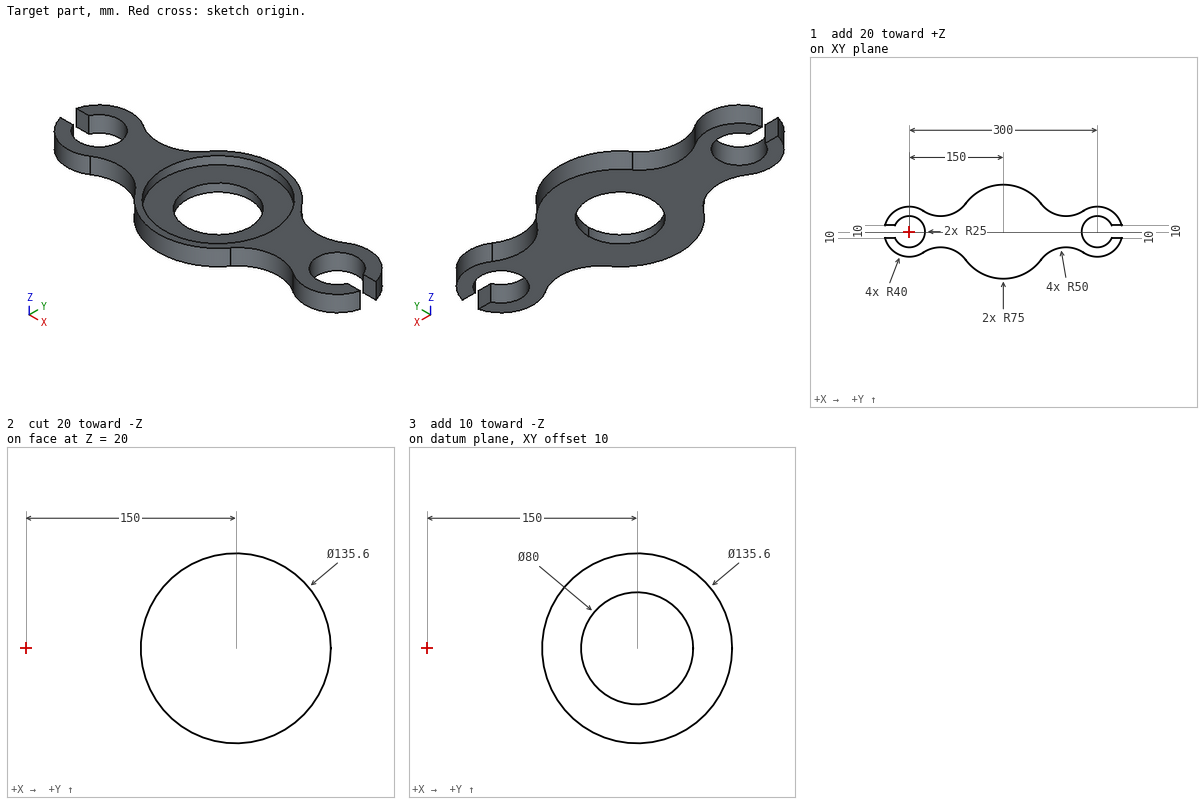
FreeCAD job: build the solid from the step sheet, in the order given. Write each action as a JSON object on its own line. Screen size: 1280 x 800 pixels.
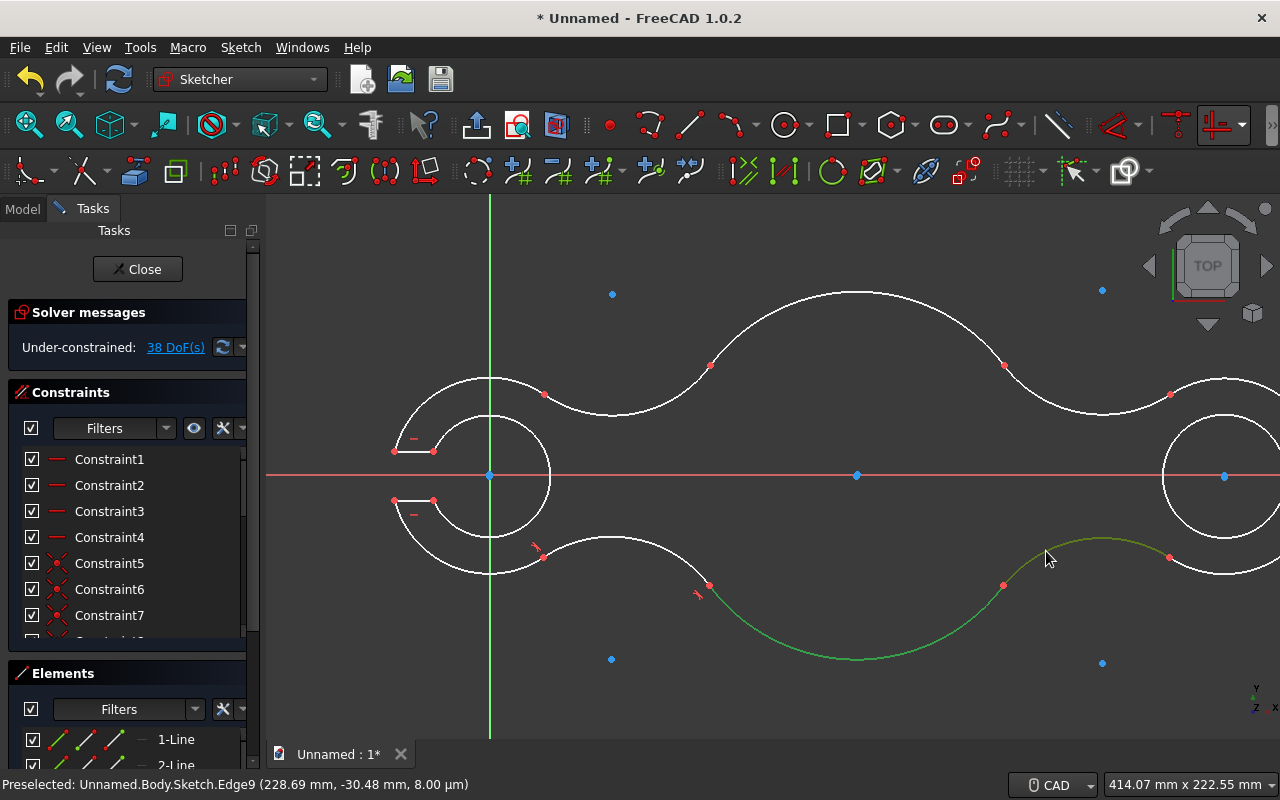
{"action": "key", "text": "t"}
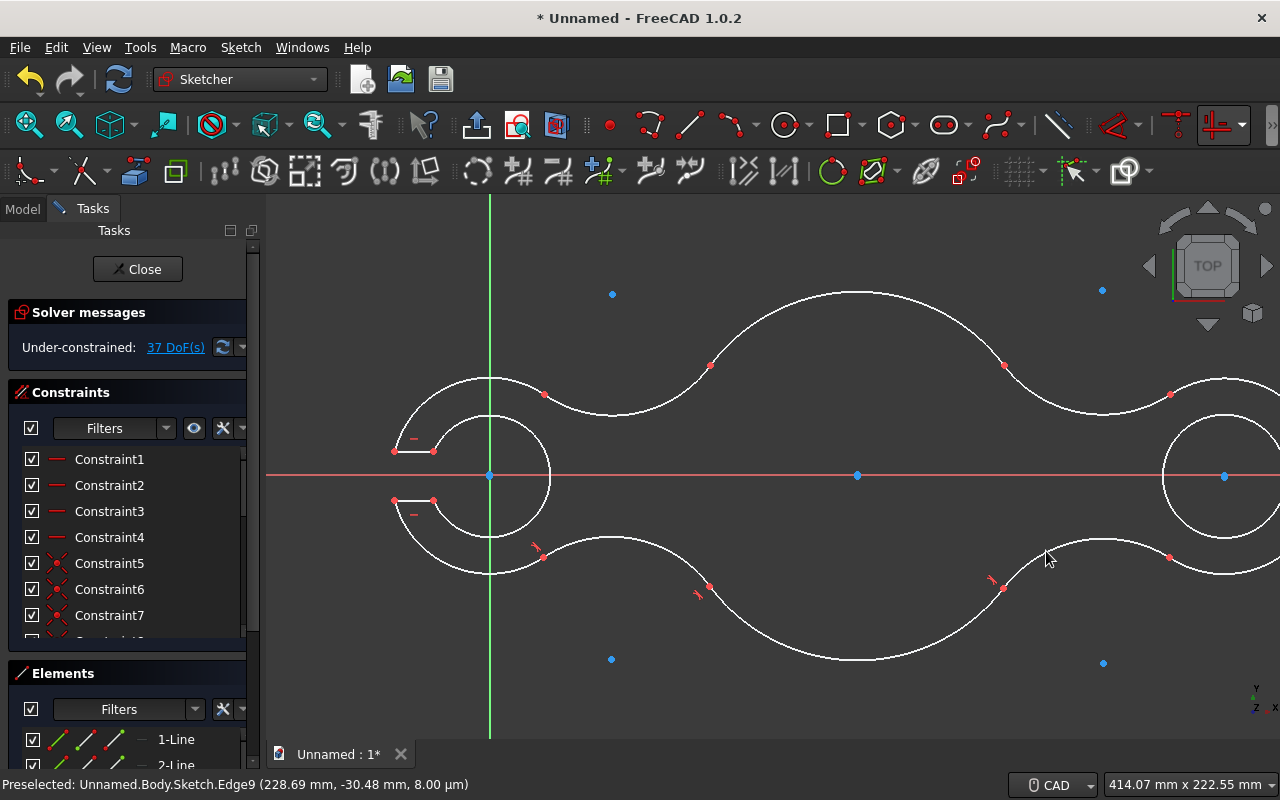
{"action": "left_click", "coordinate": [1046, 553]}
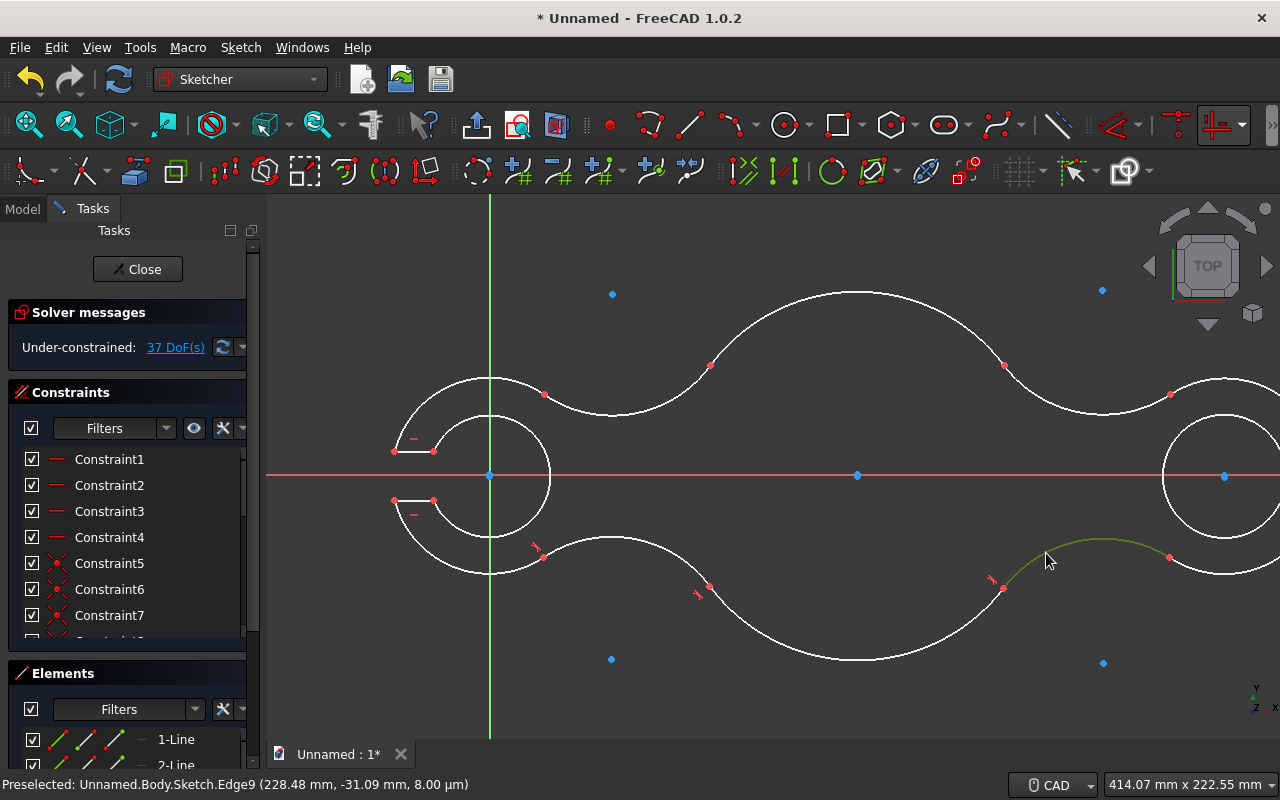
{"action": "scroll", "coordinate": [394, 449], "scroll_direction": "down", "scroll_amount": 2}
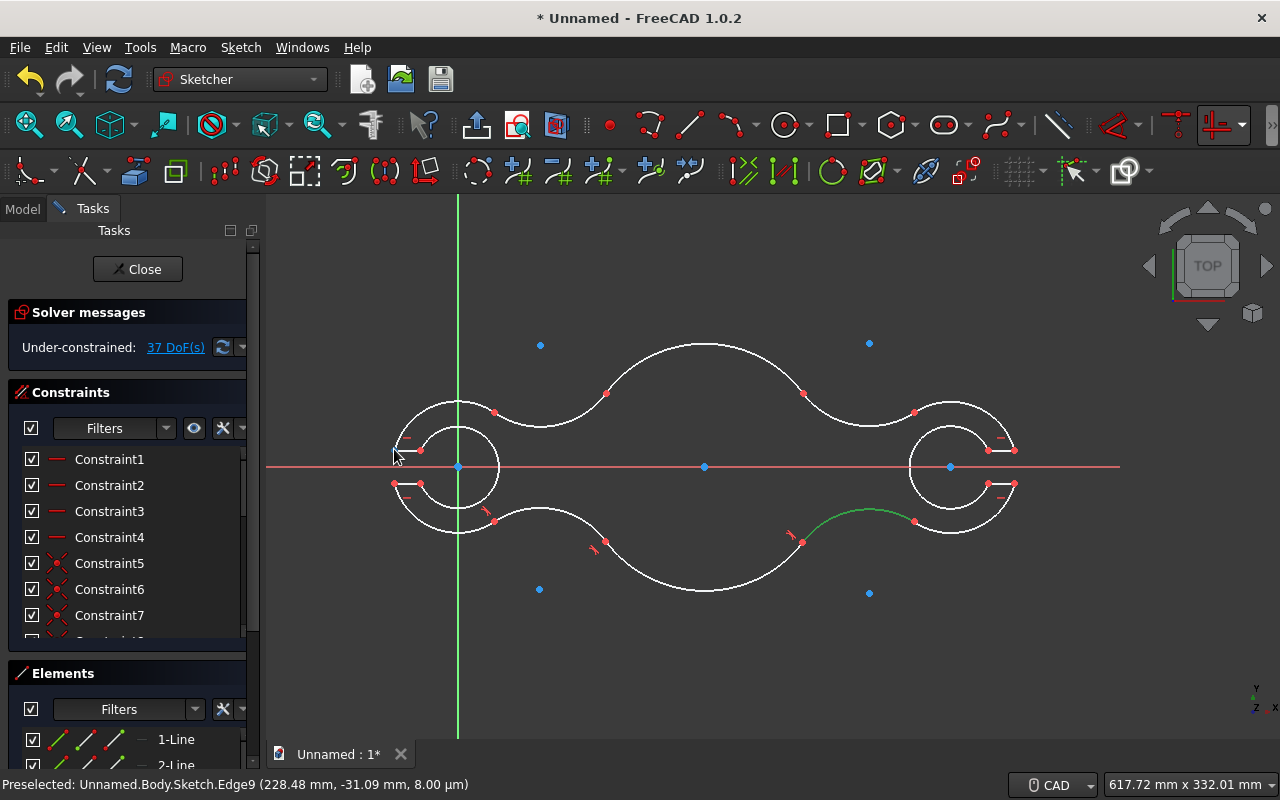
{"action": "left_click", "coordinate": [949, 533]}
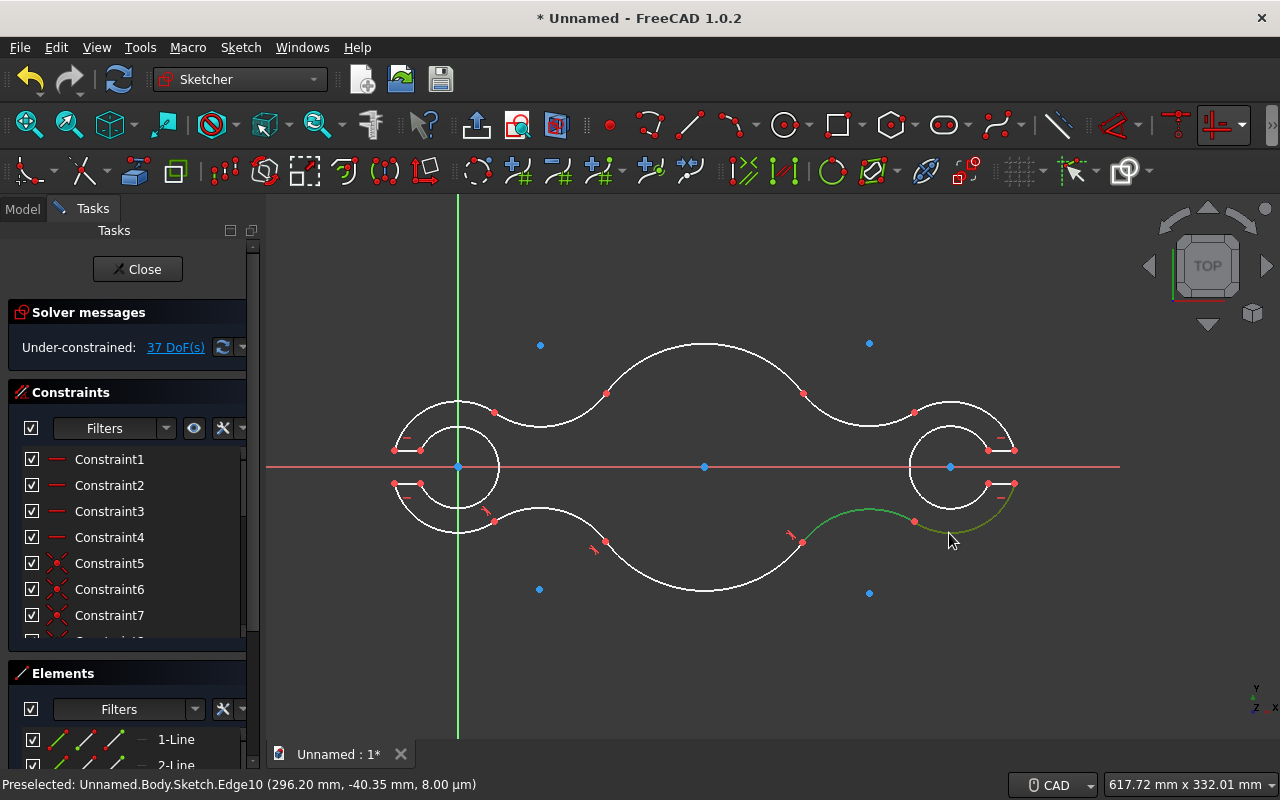
{"action": "key", "text": "t"}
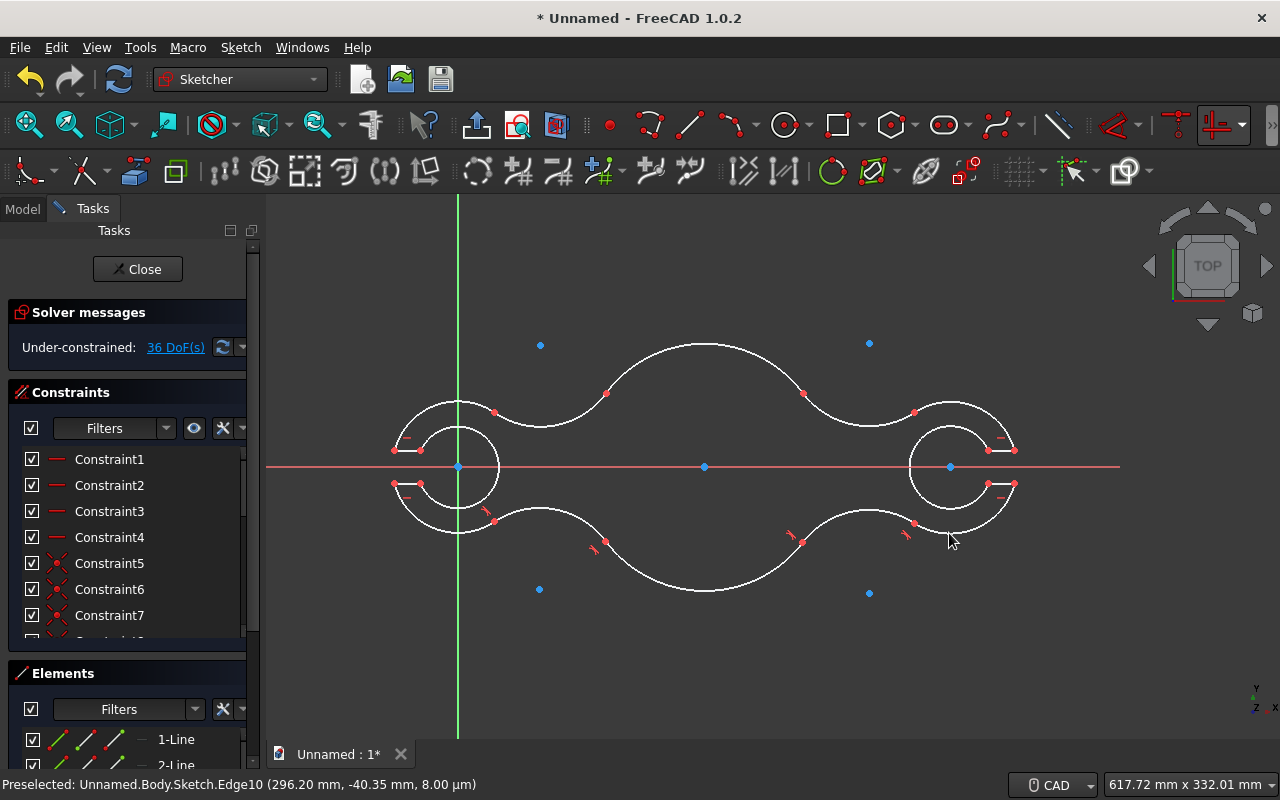
{"action": "left_click", "coordinate": [995, 419]}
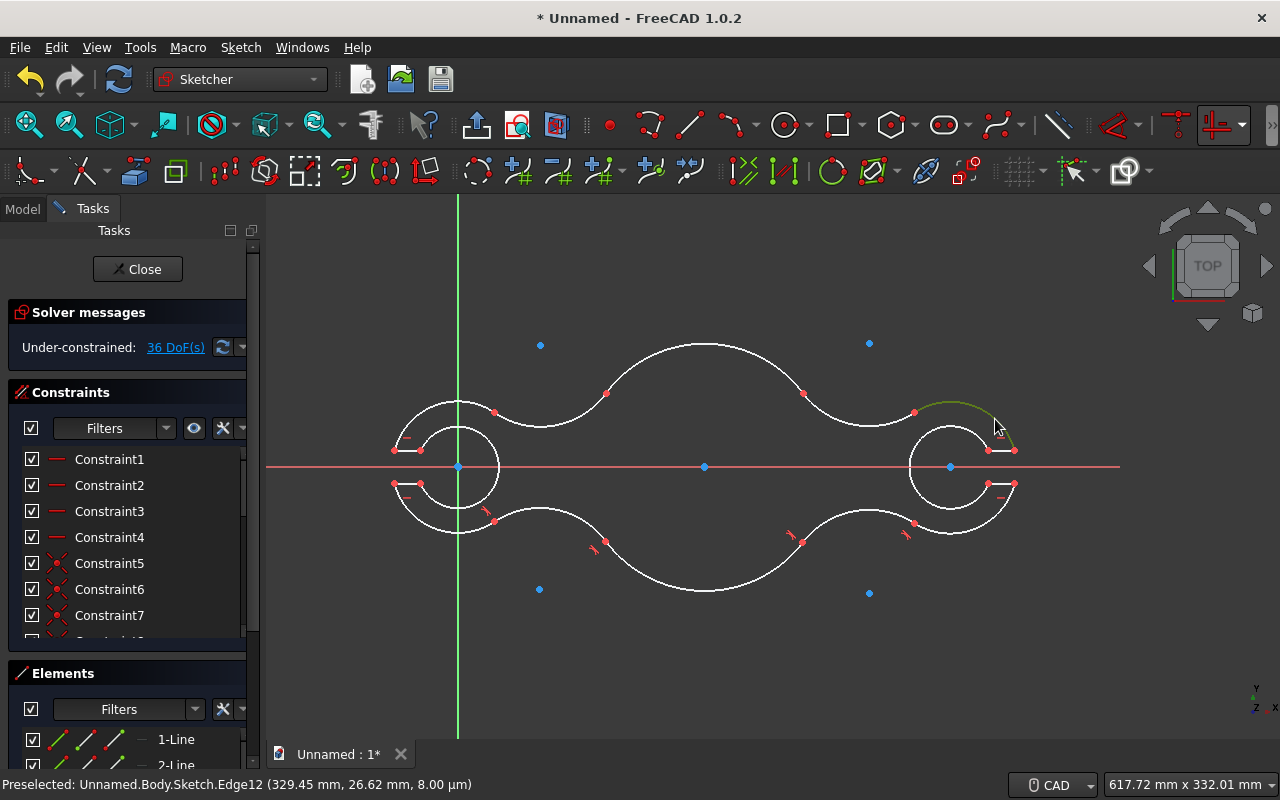
{"action": "left_click", "coordinate": [831, 417]}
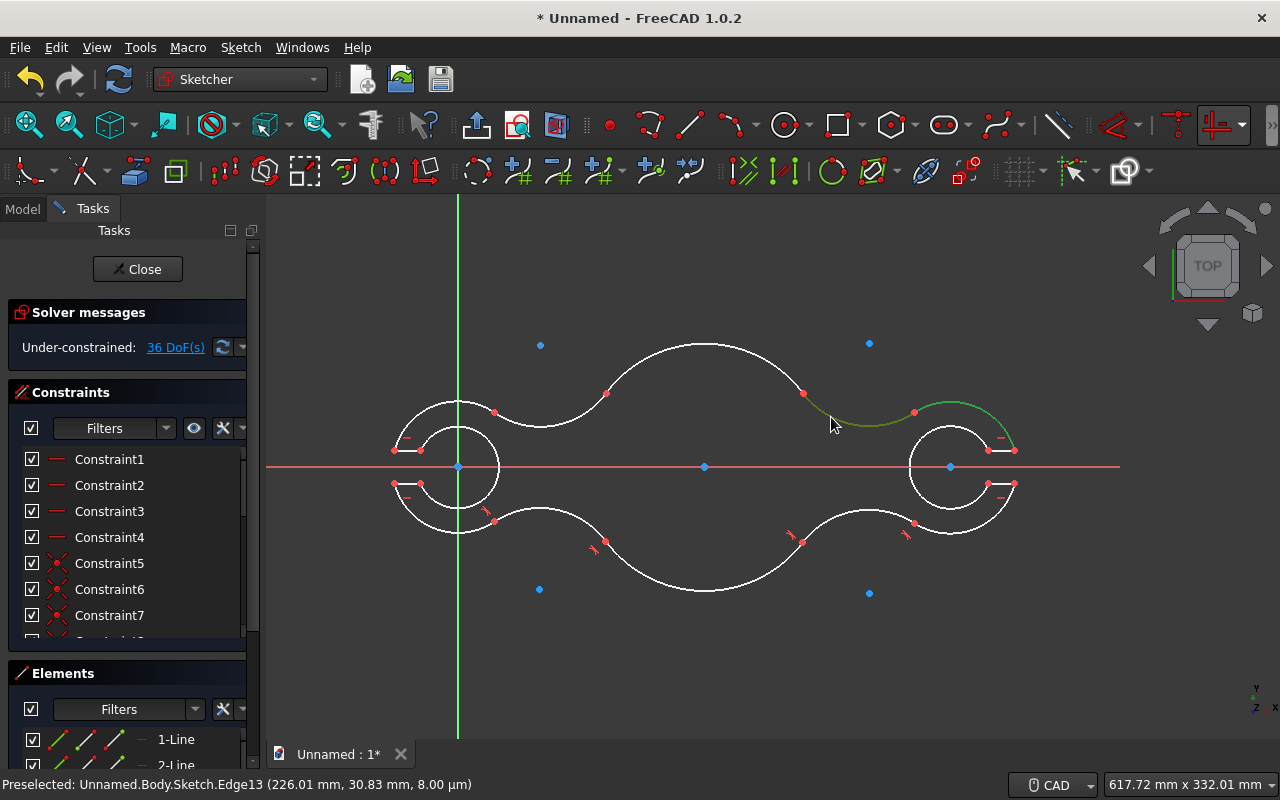
{"action": "key", "text": "t"}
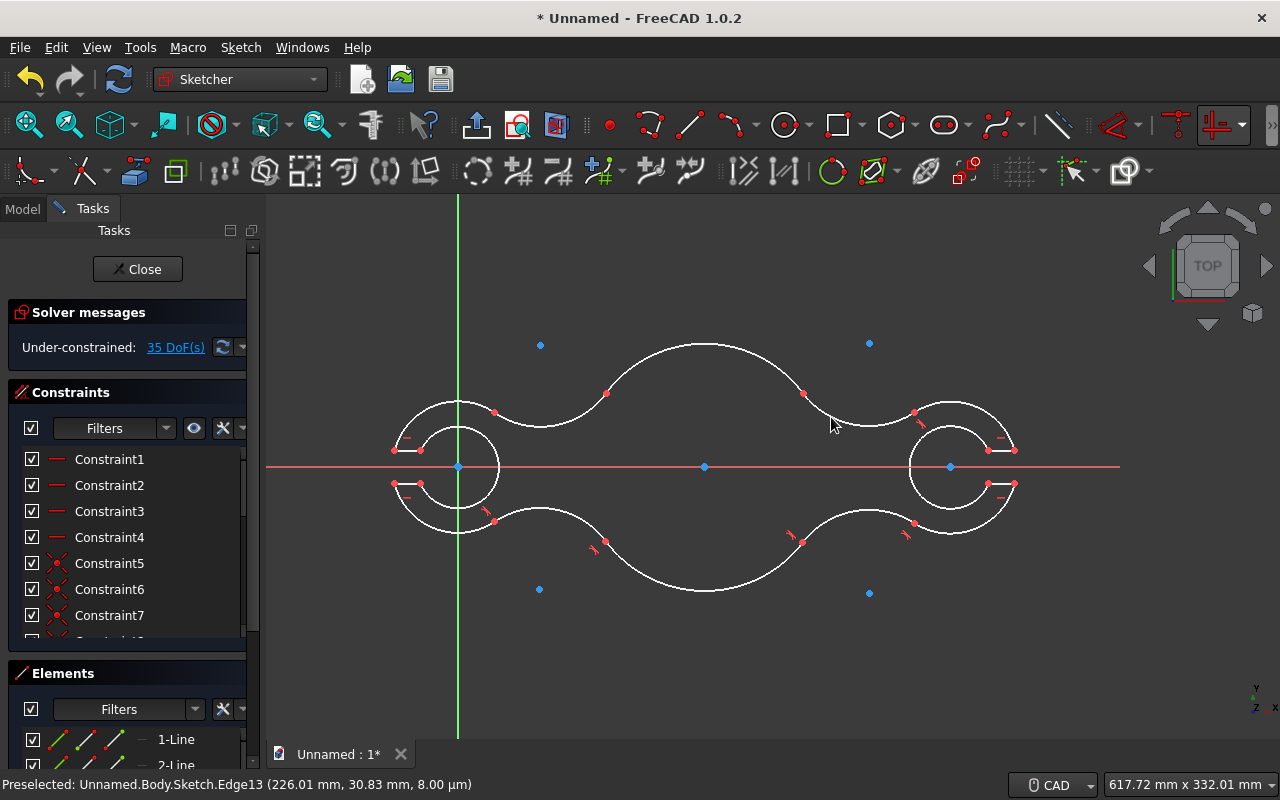
{"action": "left_click", "coordinate": [831, 417]}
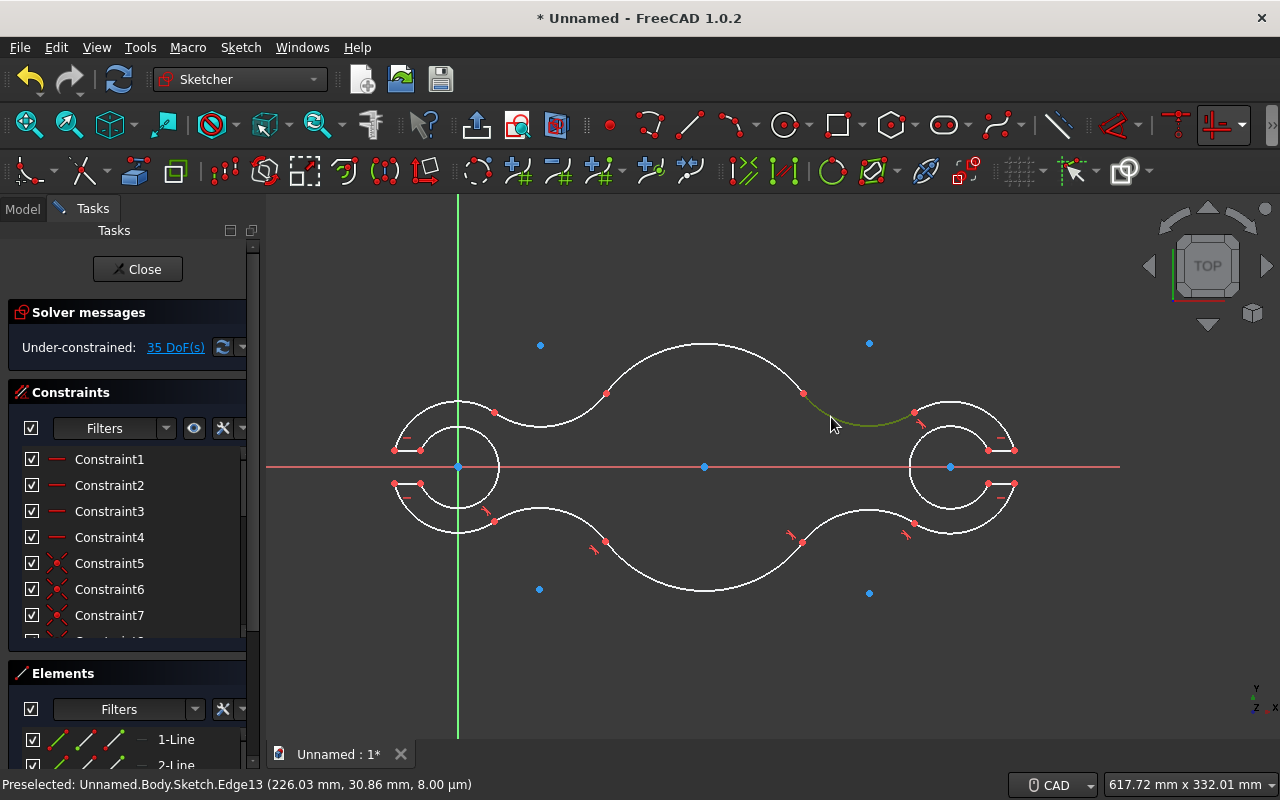
{"action": "left_click", "coordinate": [749, 352]}